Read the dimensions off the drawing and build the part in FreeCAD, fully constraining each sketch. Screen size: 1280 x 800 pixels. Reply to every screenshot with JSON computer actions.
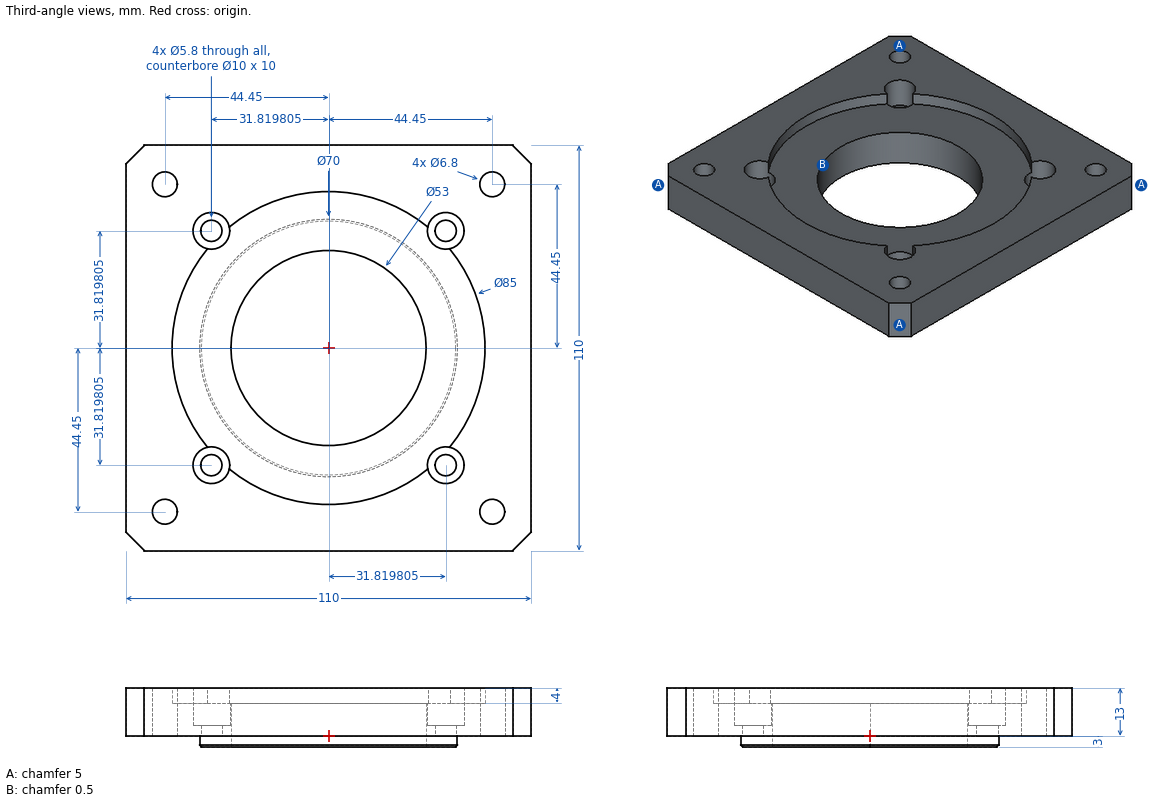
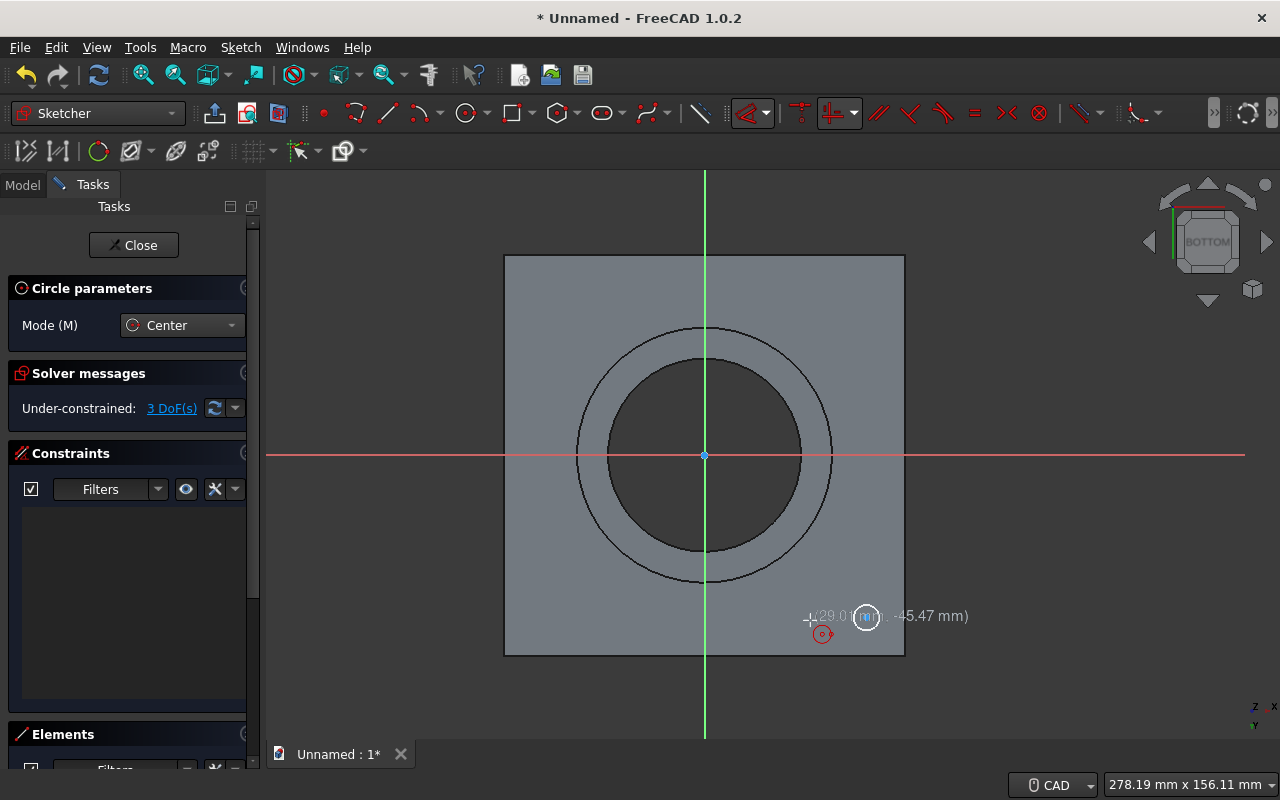
{"action": "scroll", "coordinate": [543, 617], "scroll_direction": "up", "scroll_amount": 4}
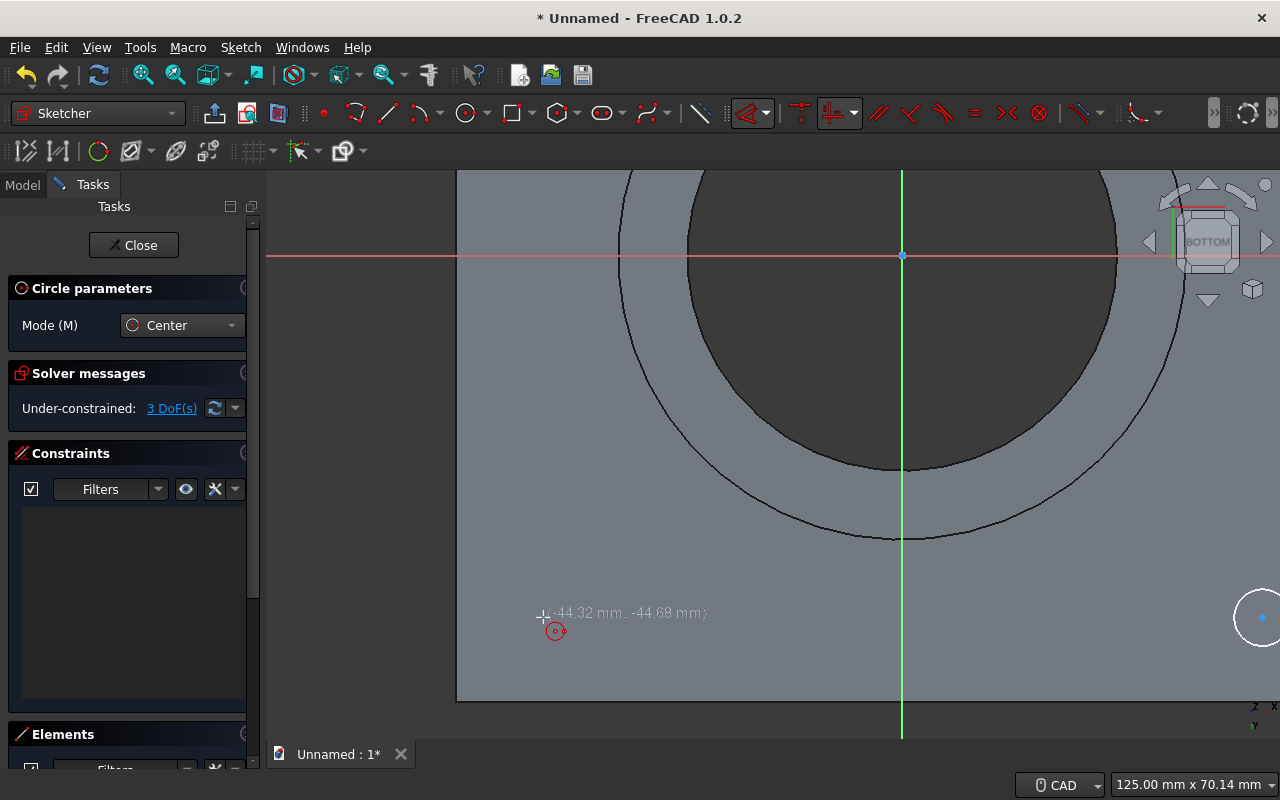
{"action": "left_click", "coordinate": [542, 616]}
{"action": "left_click", "coordinate": [561, 597]}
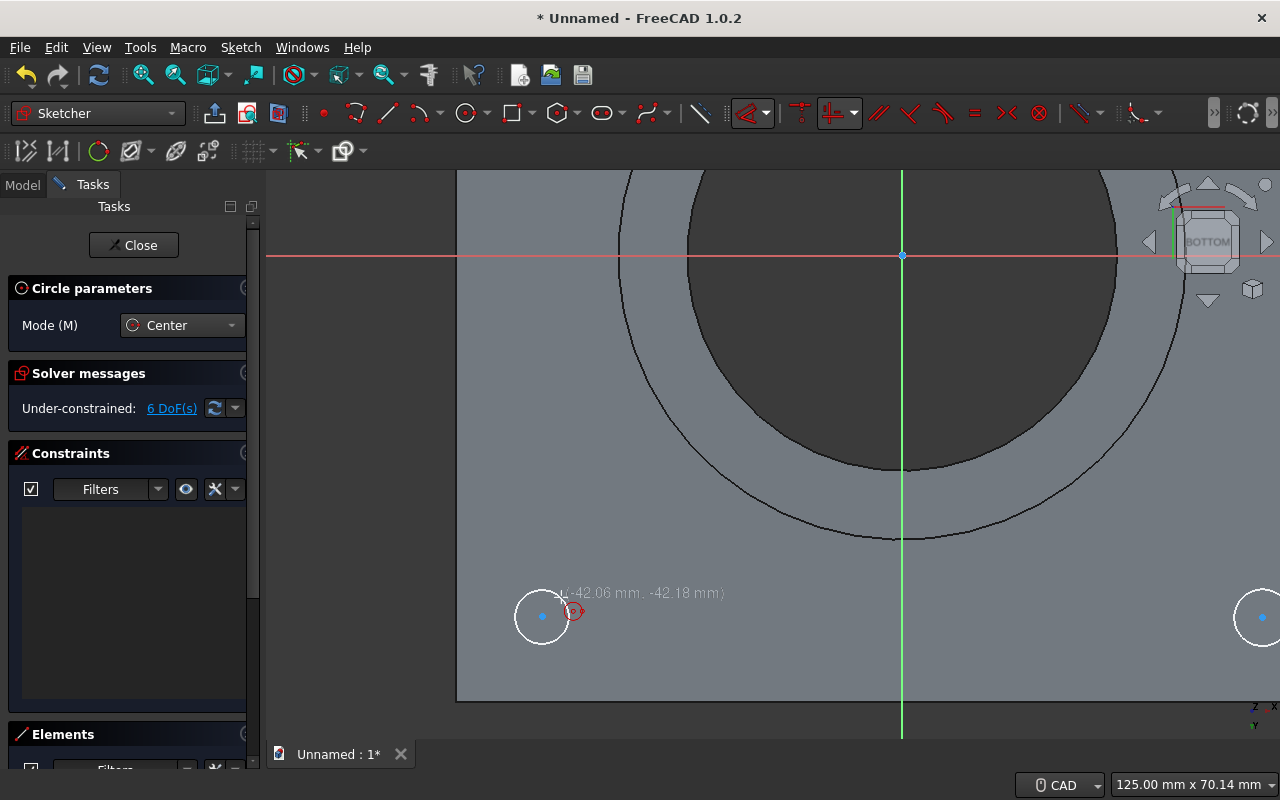
{"action": "scroll", "coordinate": [543, 617], "scroll_direction": "down", "scroll_amount": 4}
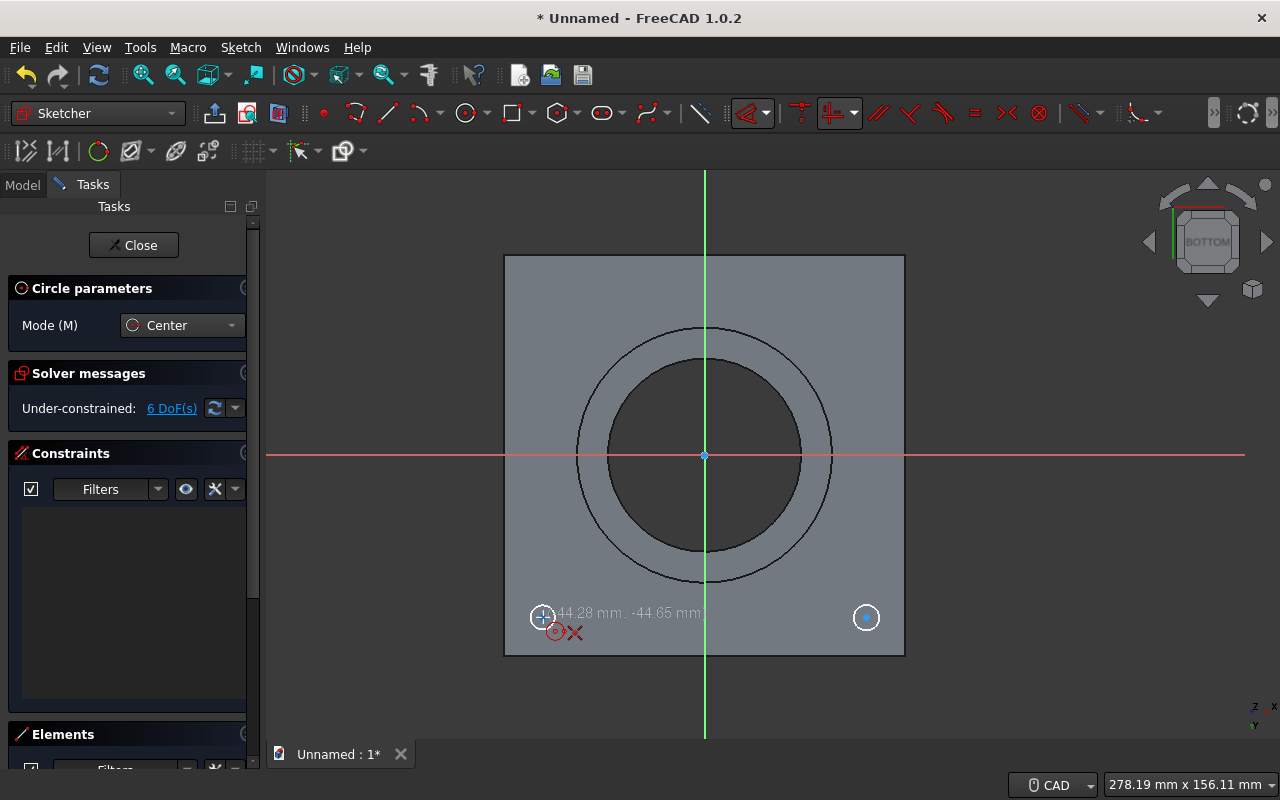
{"action": "scroll", "coordinate": [543, 293], "scroll_direction": "up", "scroll_amount": 4}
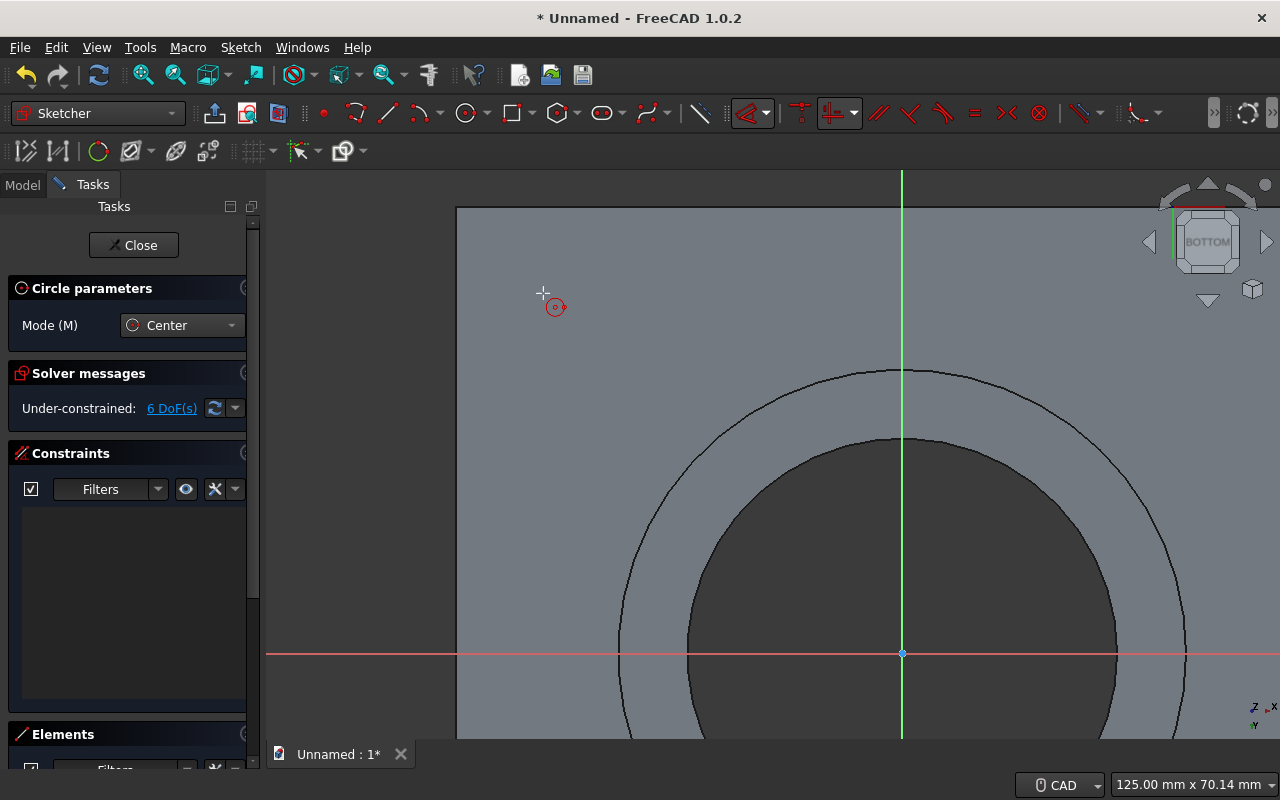
{"action": "left_click", "coordinate": [542, 293]}
{"action": "left_click", "coordinate": [561, 274]}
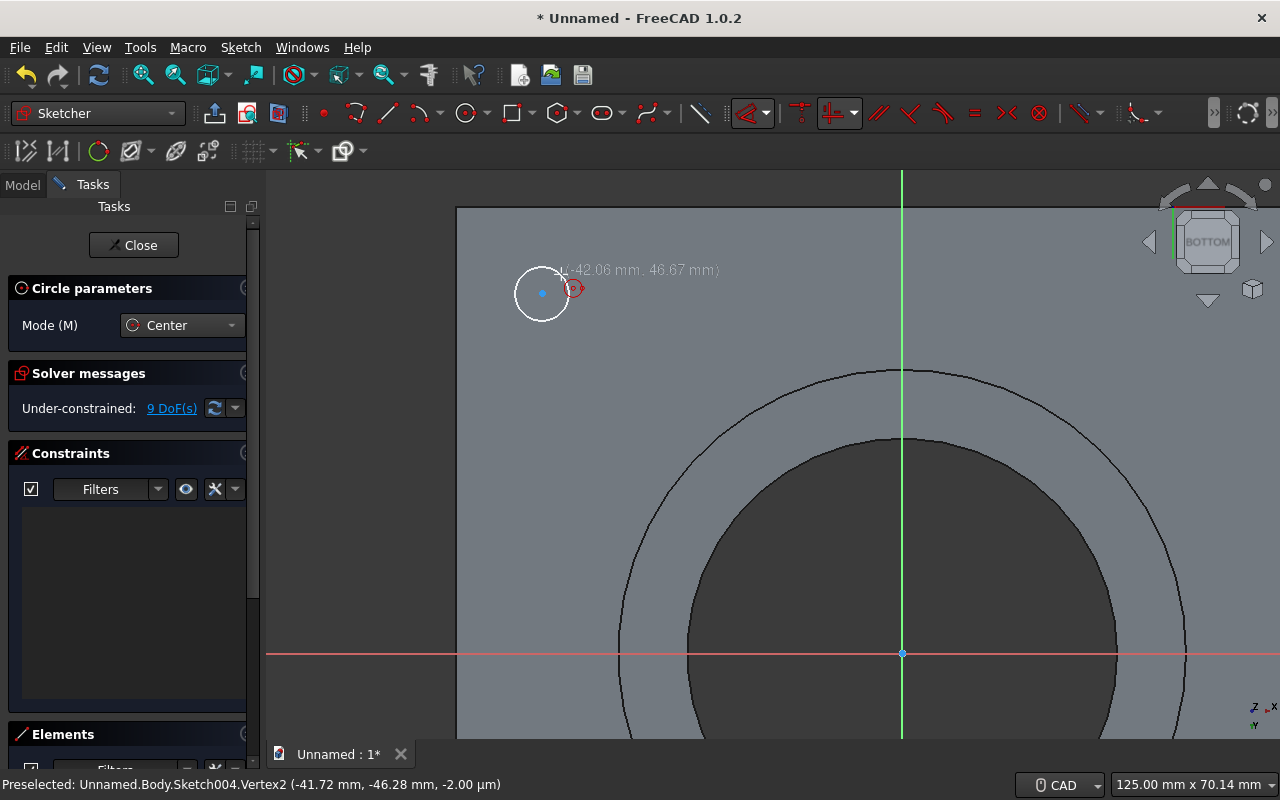
{"action": "scroll", "coordinate": [543, 292], "scroll_direction": "down", "scroll_amount": 4}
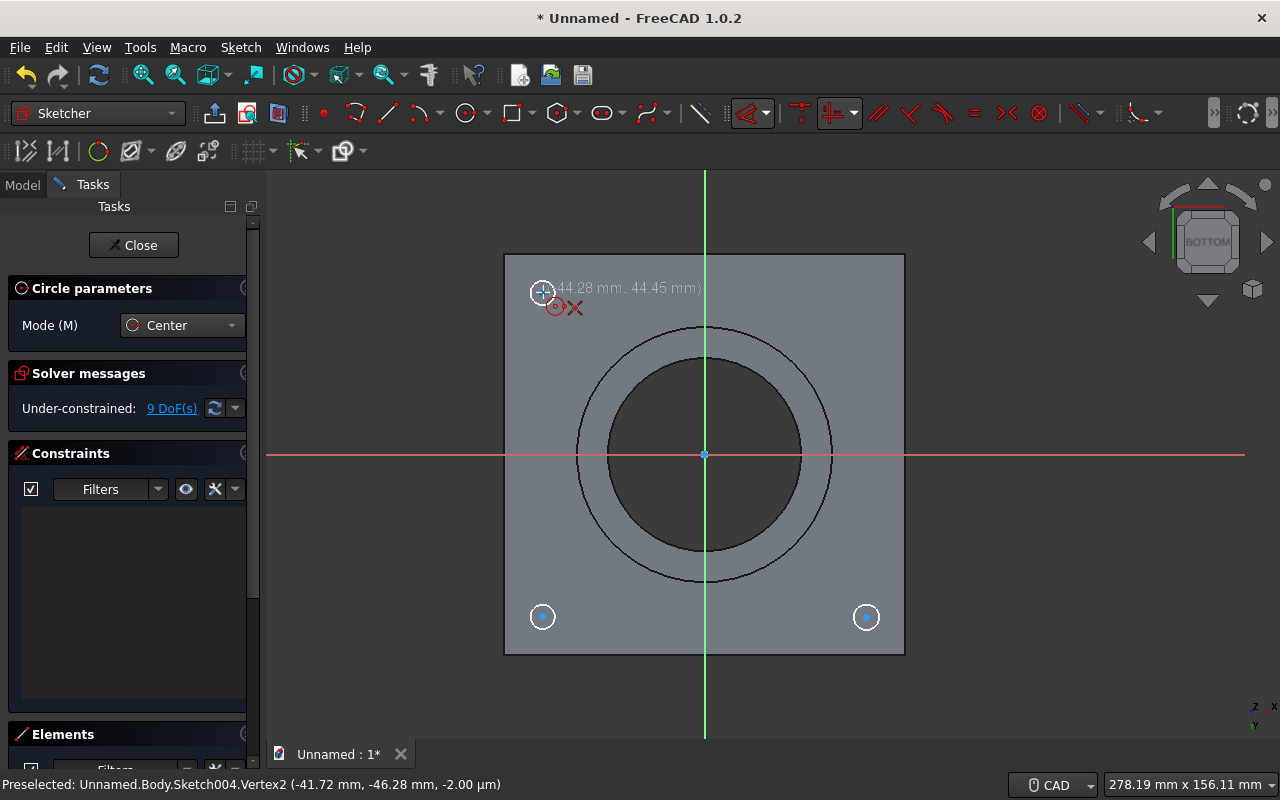
{"action": "scroll", "coordinate": [867, 293], "scroll_direction": "up", "scroll_amount": 4}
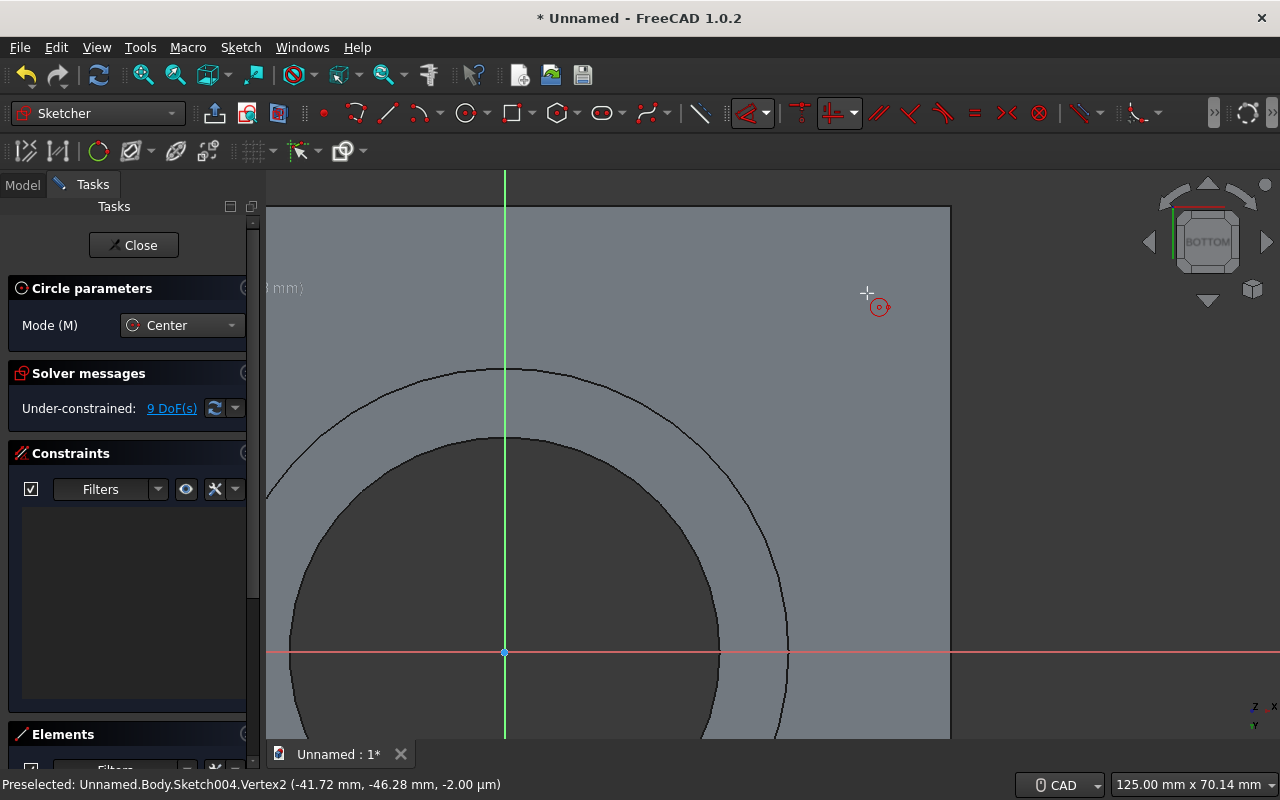
{"action": "left_click", "coordinate": [865, 292]}
{"action": "left_click", "coordinate": [885, 272]}
{"action": "key", "text": "Escape"}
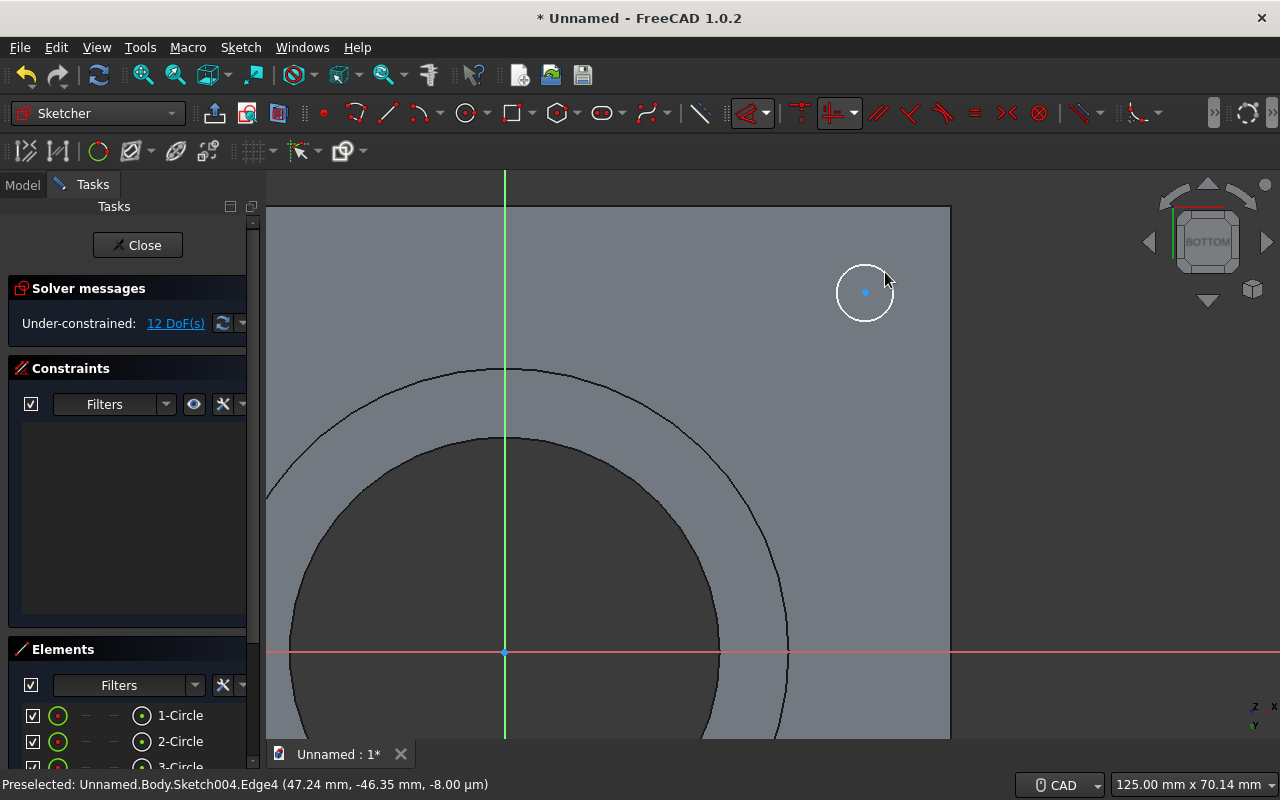
{"action": "scroll", "coordinate": [868, 293], "scroll_direction": "down", "scroll_amount": 4}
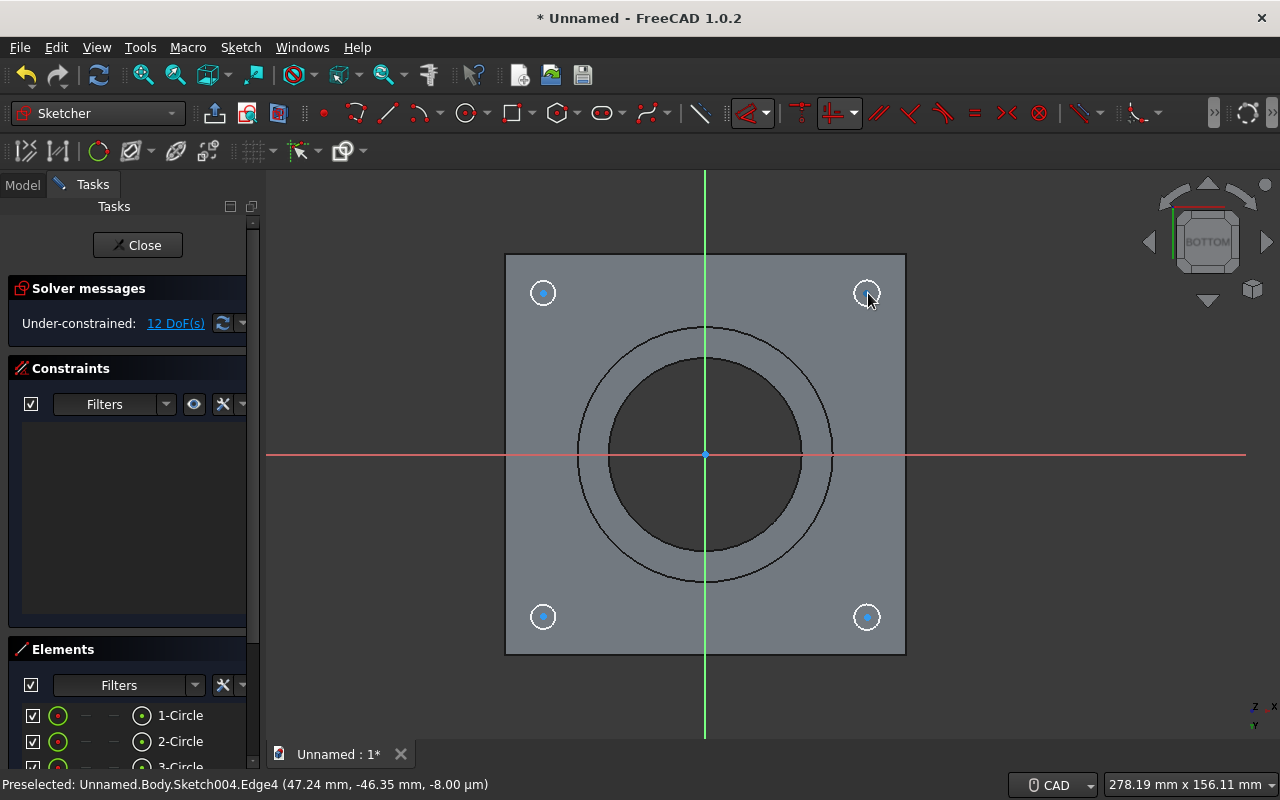
{"action": "left_click", "coordinate": [876, 608]}